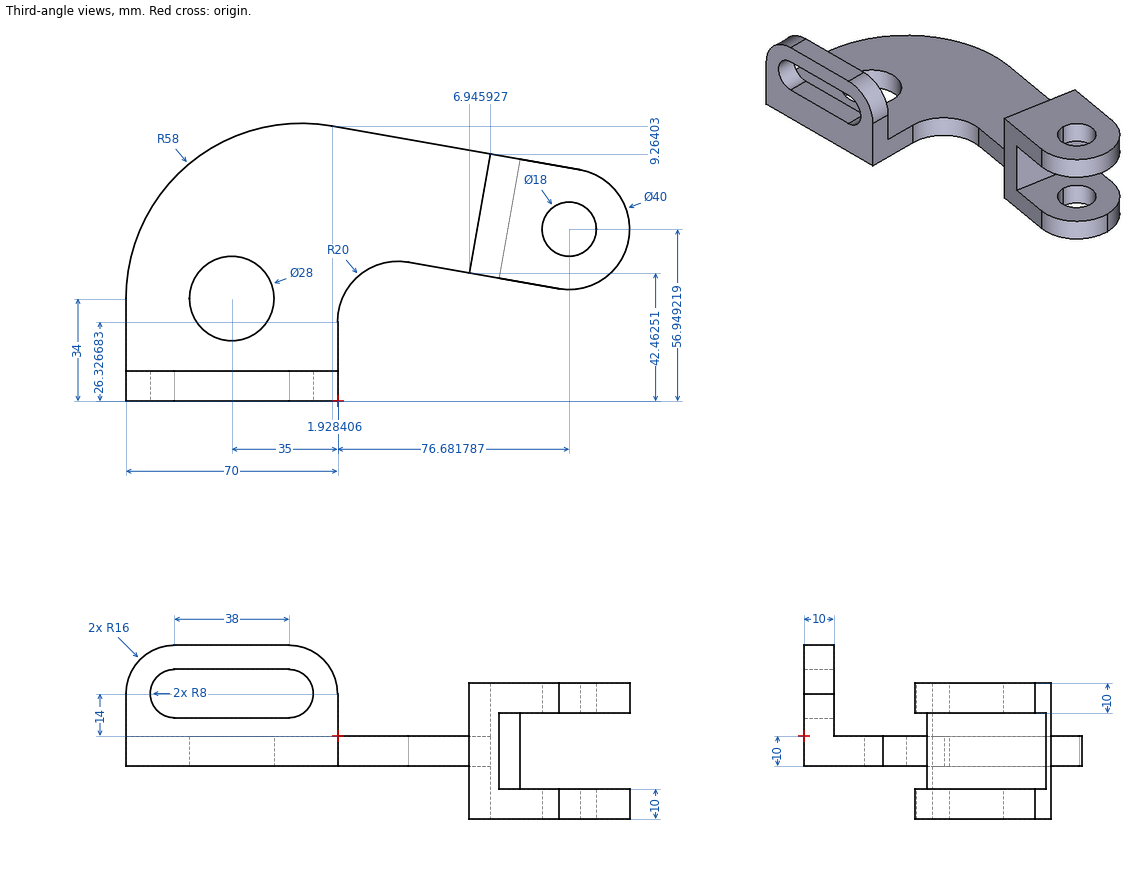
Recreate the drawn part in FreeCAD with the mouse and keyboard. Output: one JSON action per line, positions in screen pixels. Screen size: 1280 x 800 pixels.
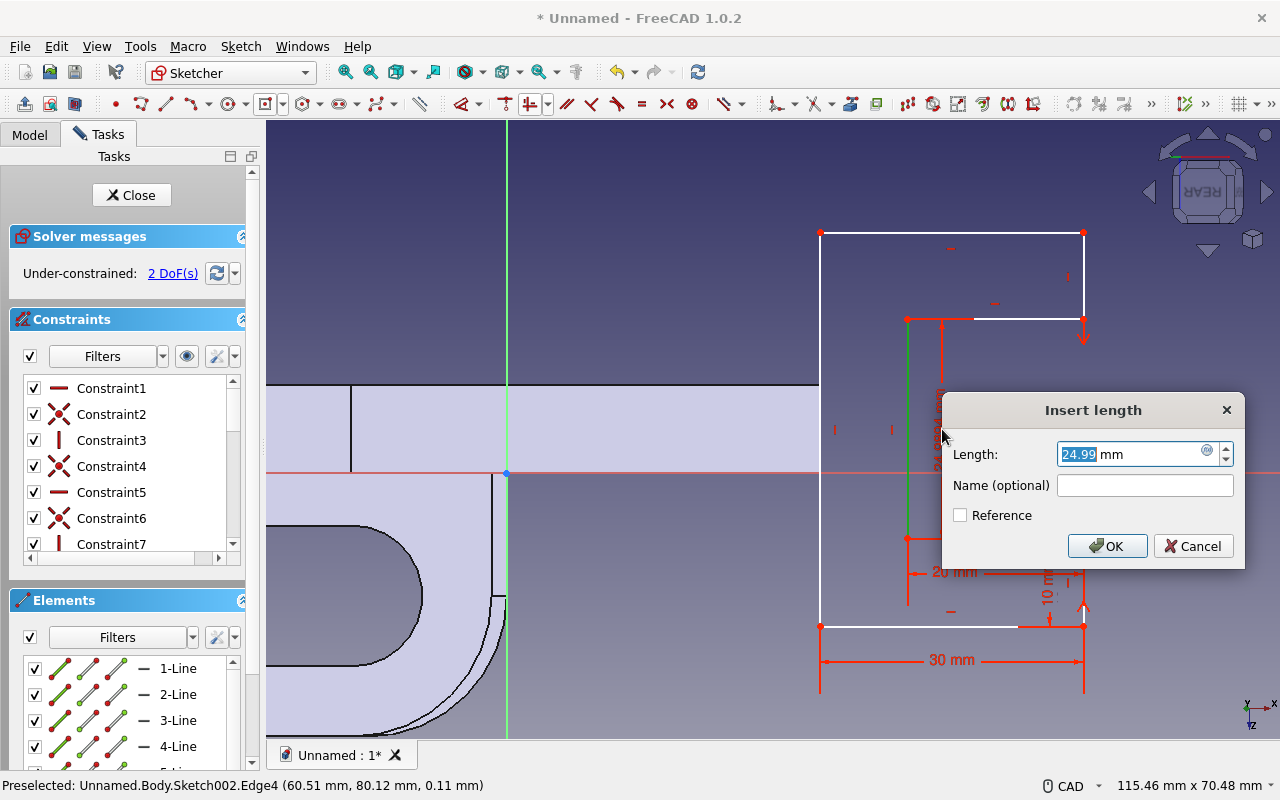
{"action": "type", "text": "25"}
{"action": "key", "text": "Return"}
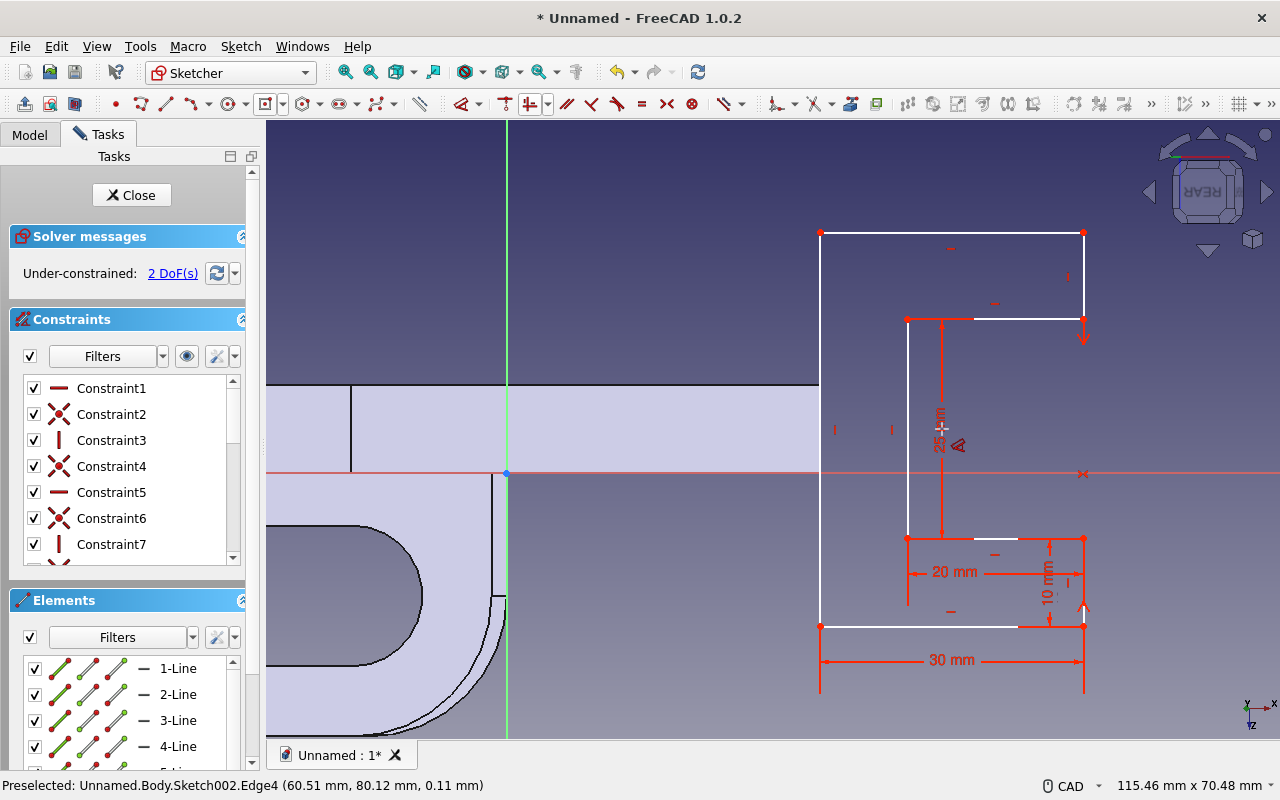
{"action": "left_click", "coordinate": [1084, 293]}
{"action": "left_click", "coordinate": [1050, 276]}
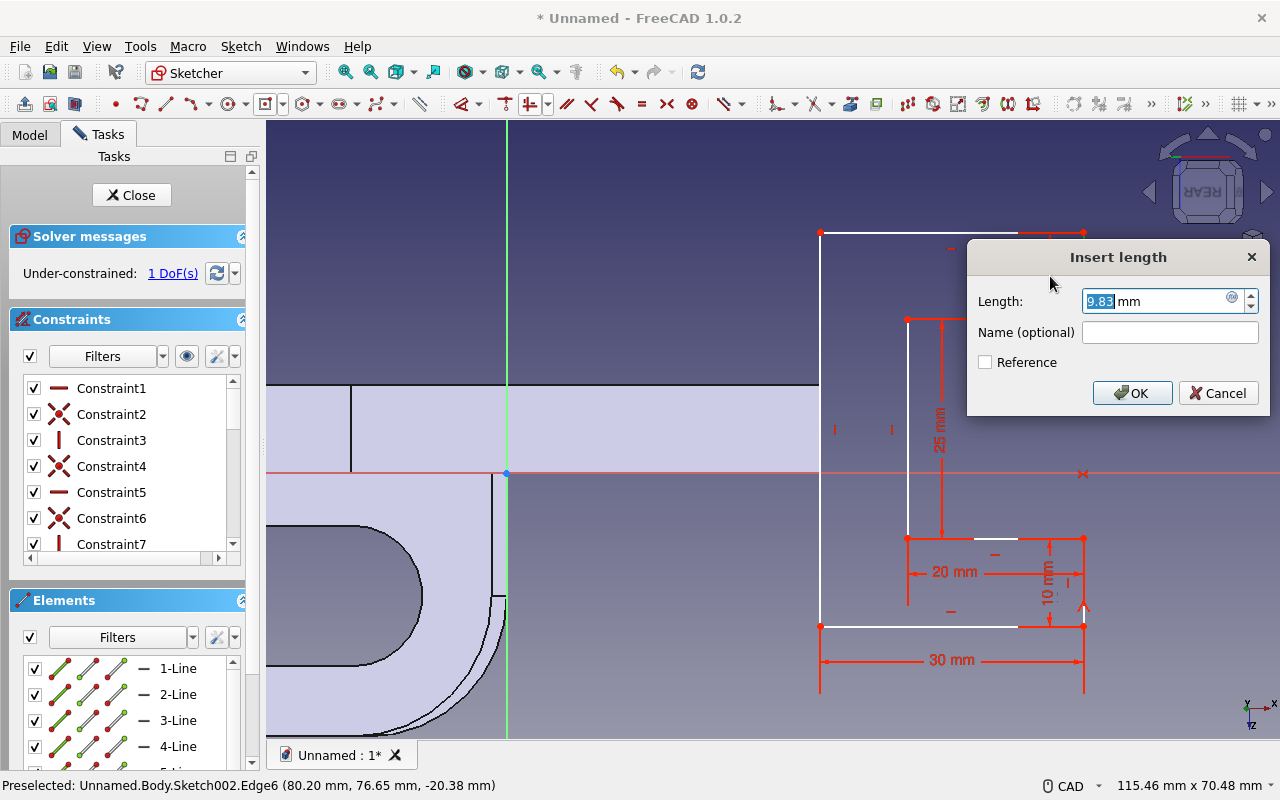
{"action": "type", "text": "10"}
{"action": "key", "text": "Return"}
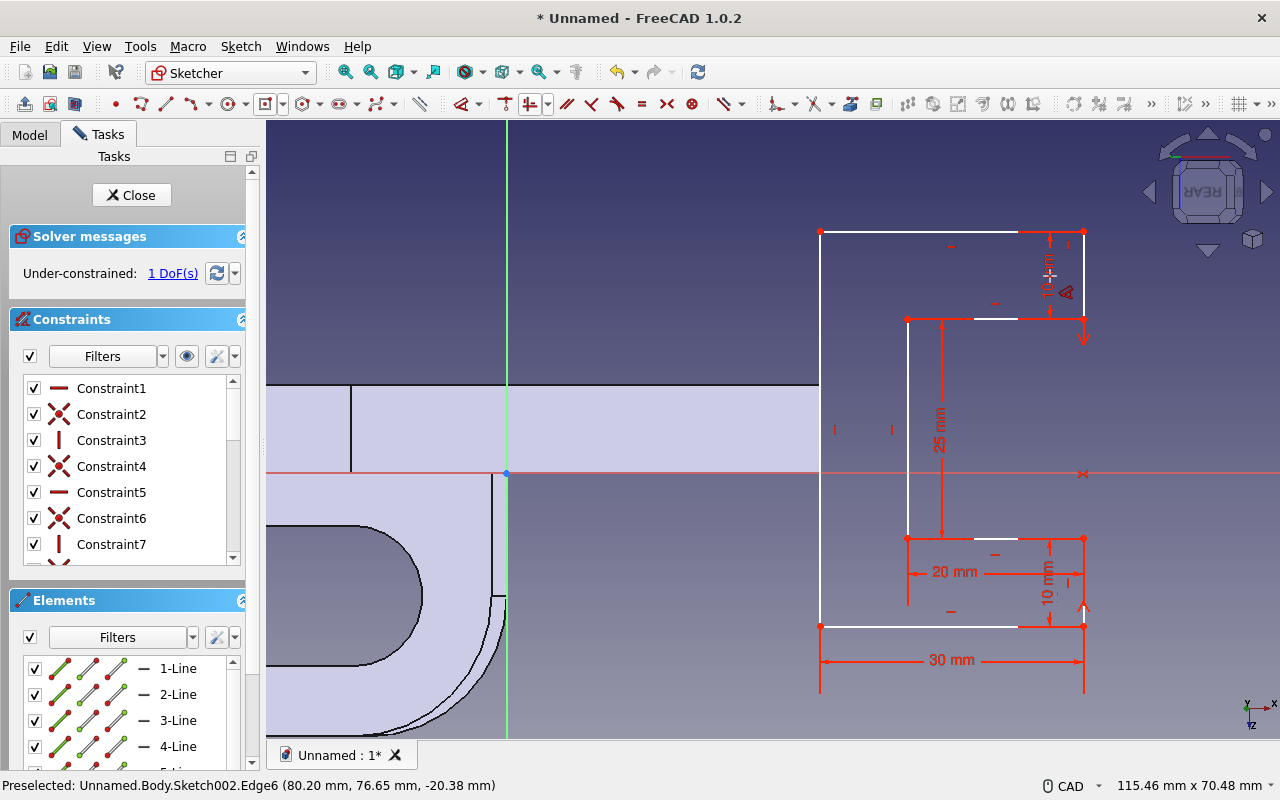
{"action": "left_click", "coordinate": [820, 627]}
{"action": "left_click", "coordinate": [663, 661]}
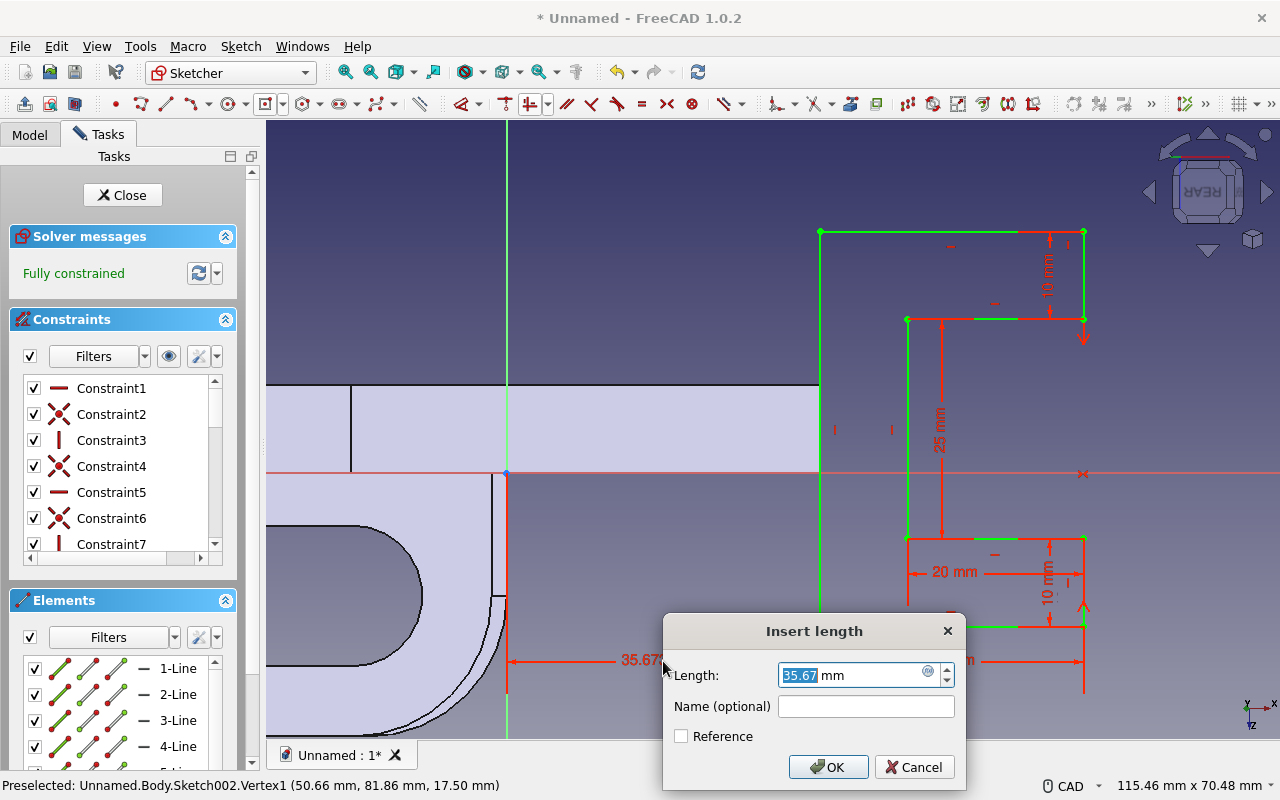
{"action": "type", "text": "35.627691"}
{"action": "key", "text": "Return"}
{"action": "key", "text": "Escape"}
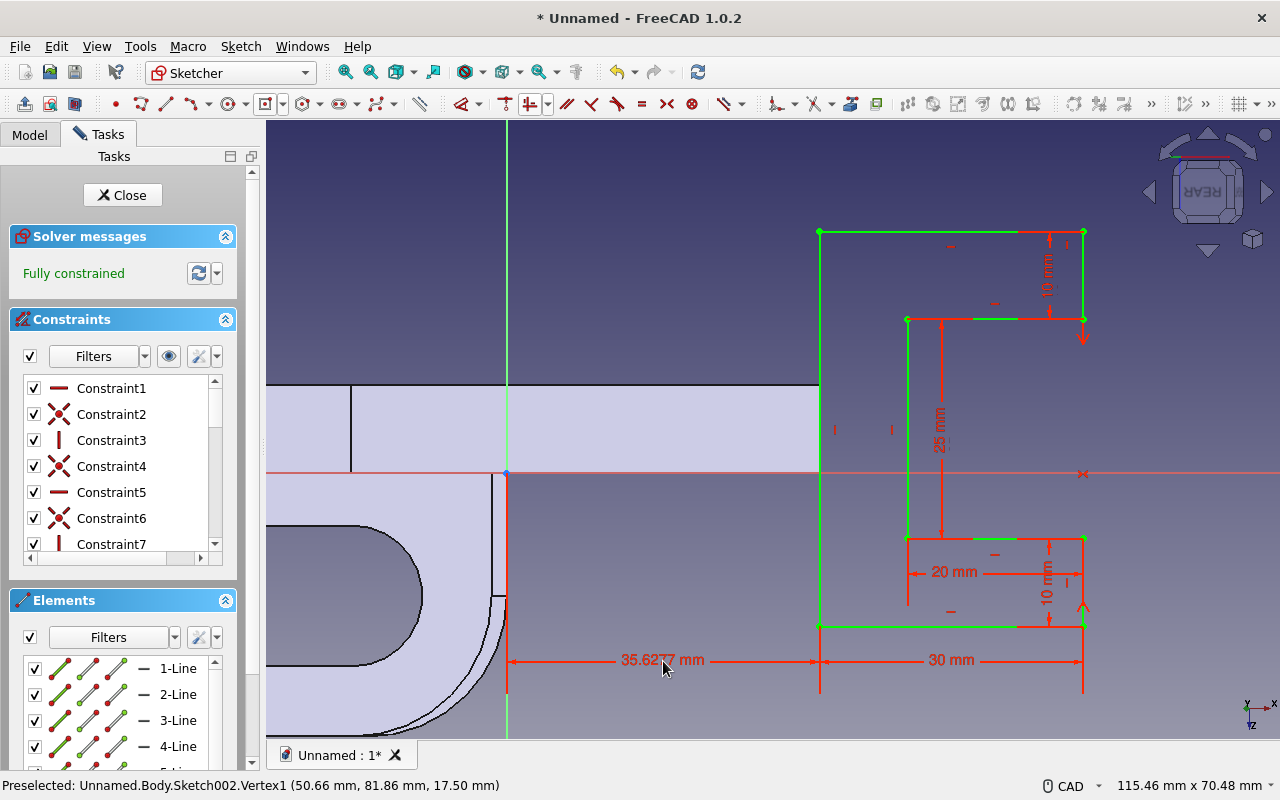
{"action": "left_click", "coordinate": [123, 195]}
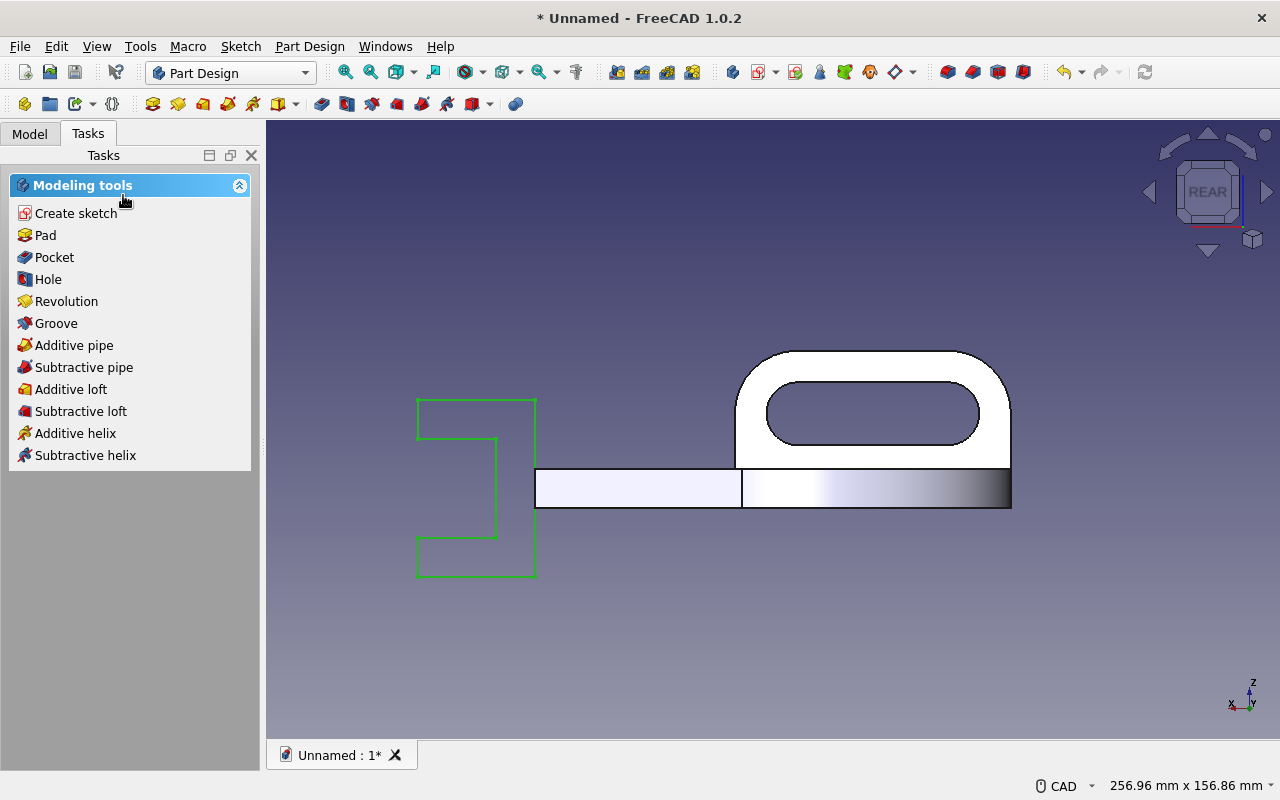
{"action": "left_click", "coordinate": [153, 104]}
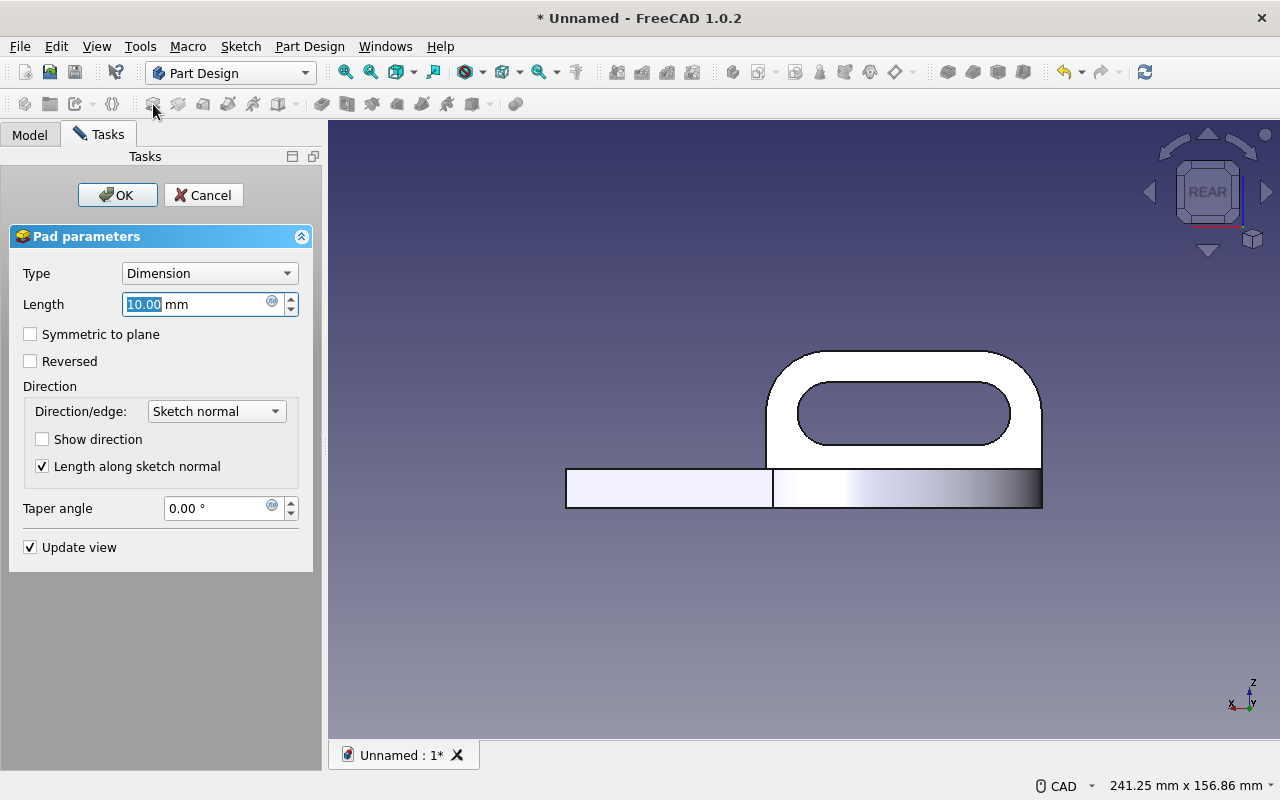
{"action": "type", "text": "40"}
{"action": "key", "text": "Tab"}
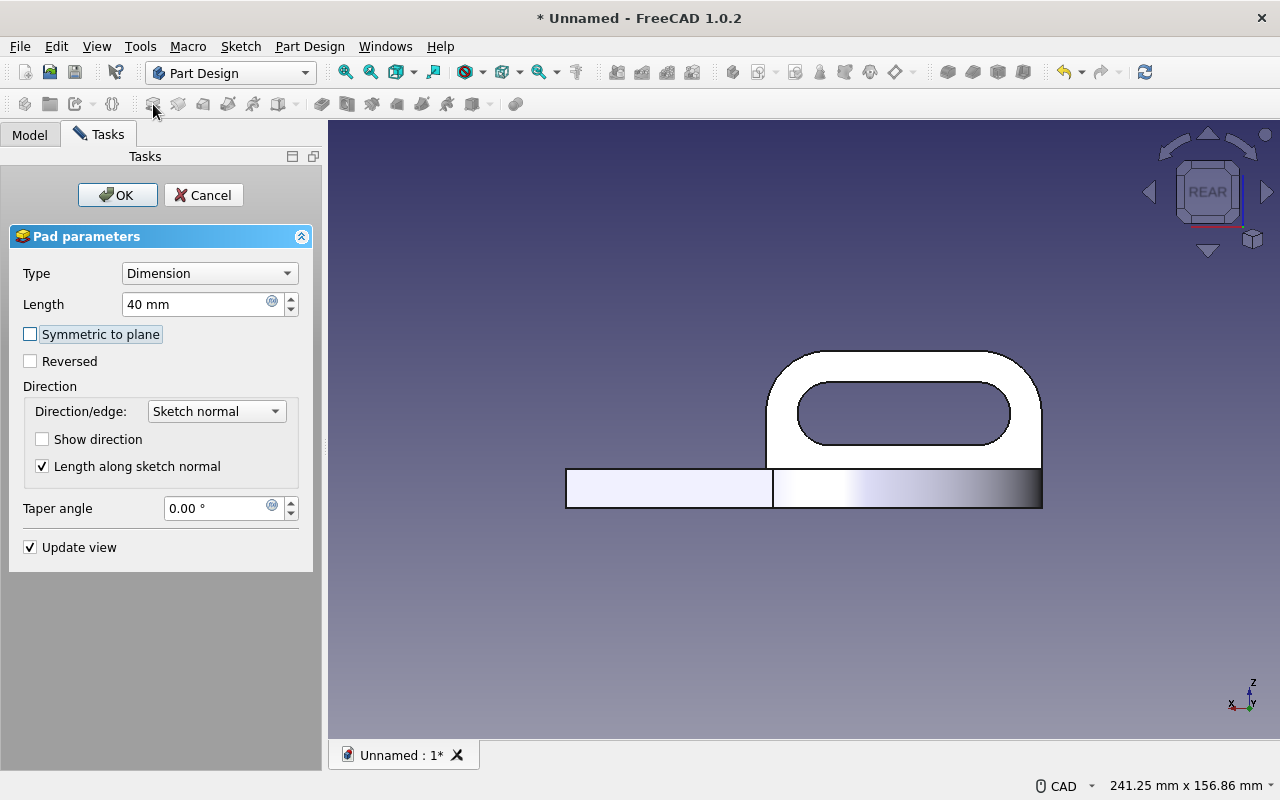
{"action": "left_click", "coordinate": [31, 361]}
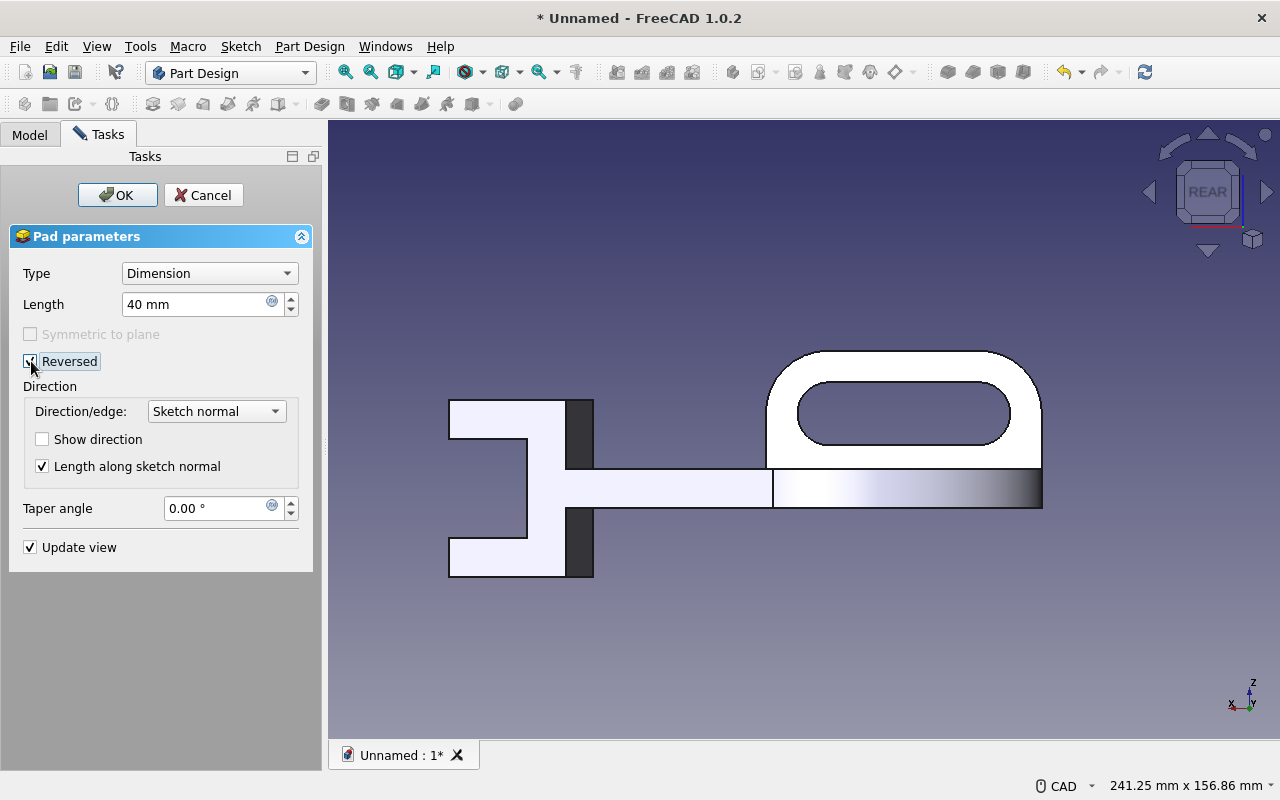
{"action": "left_click", "coordinate": [118, 195]}